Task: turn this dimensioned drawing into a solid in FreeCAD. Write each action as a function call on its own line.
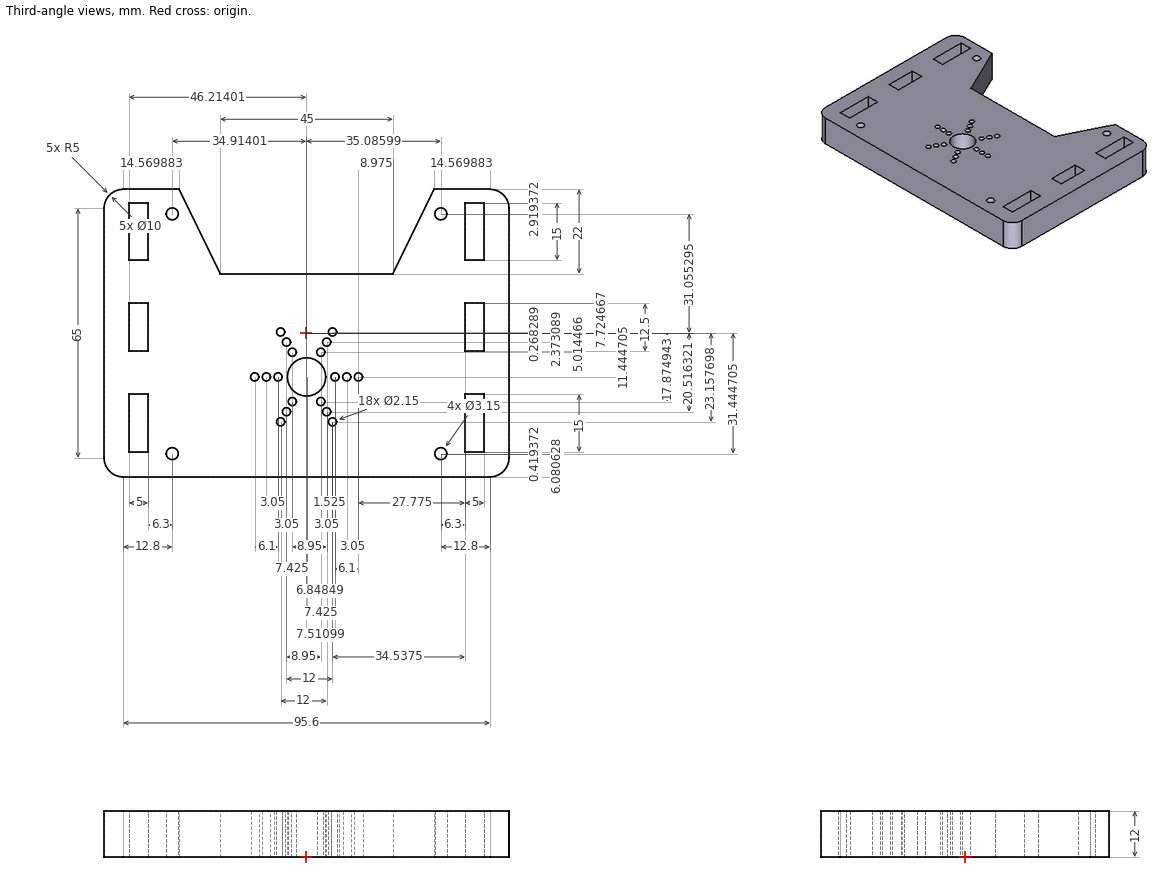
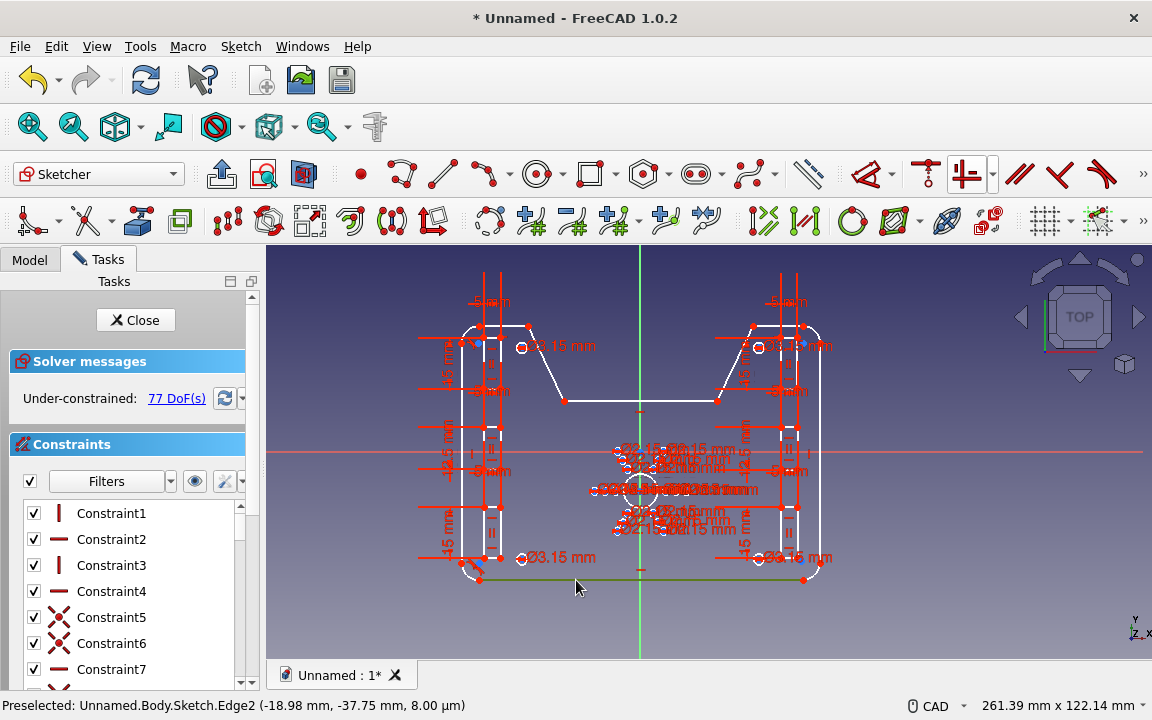
click(815, 575)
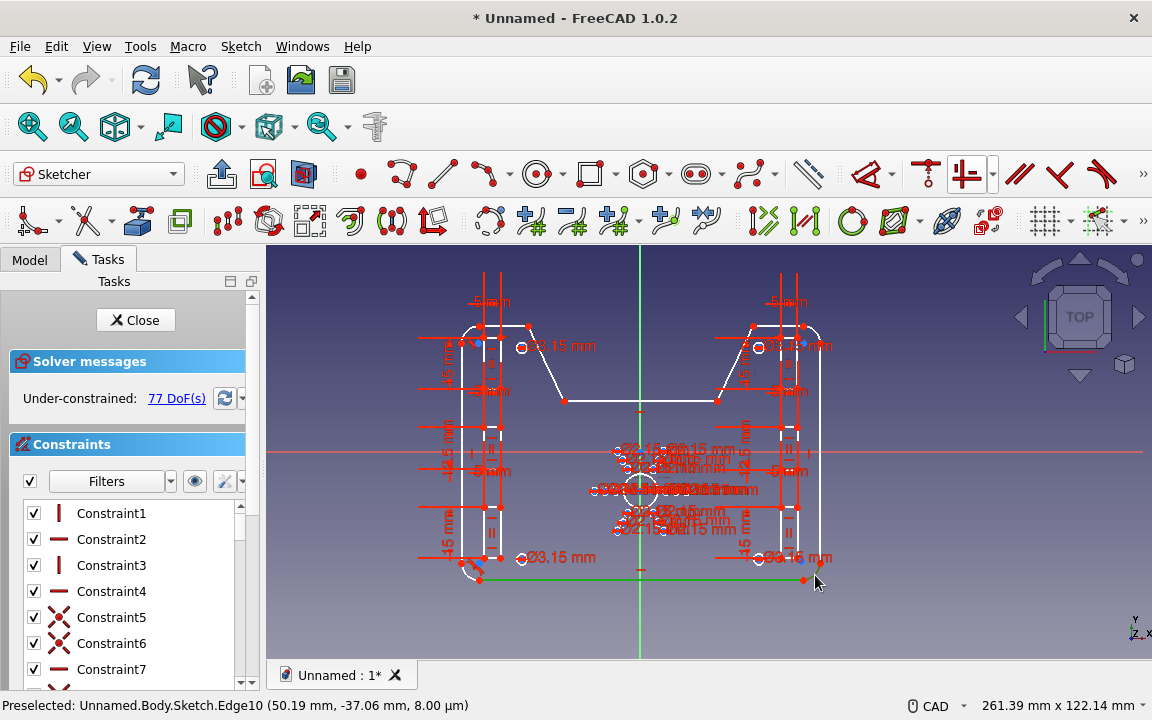
key(t)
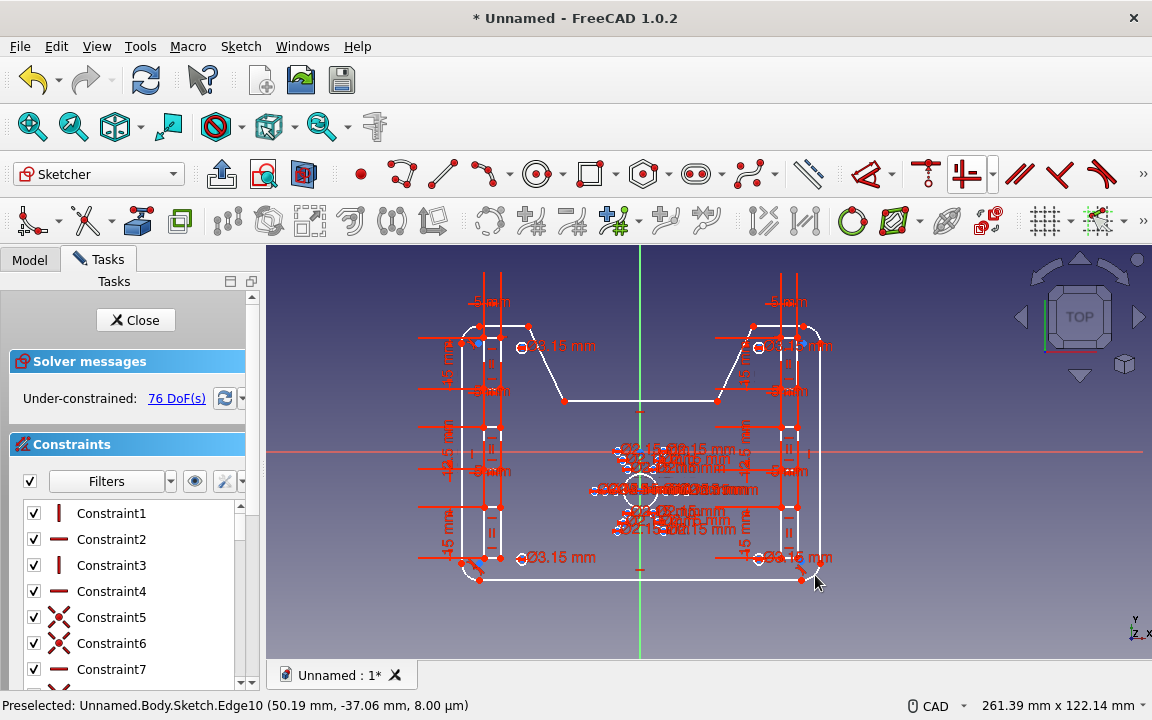
click(820, 497)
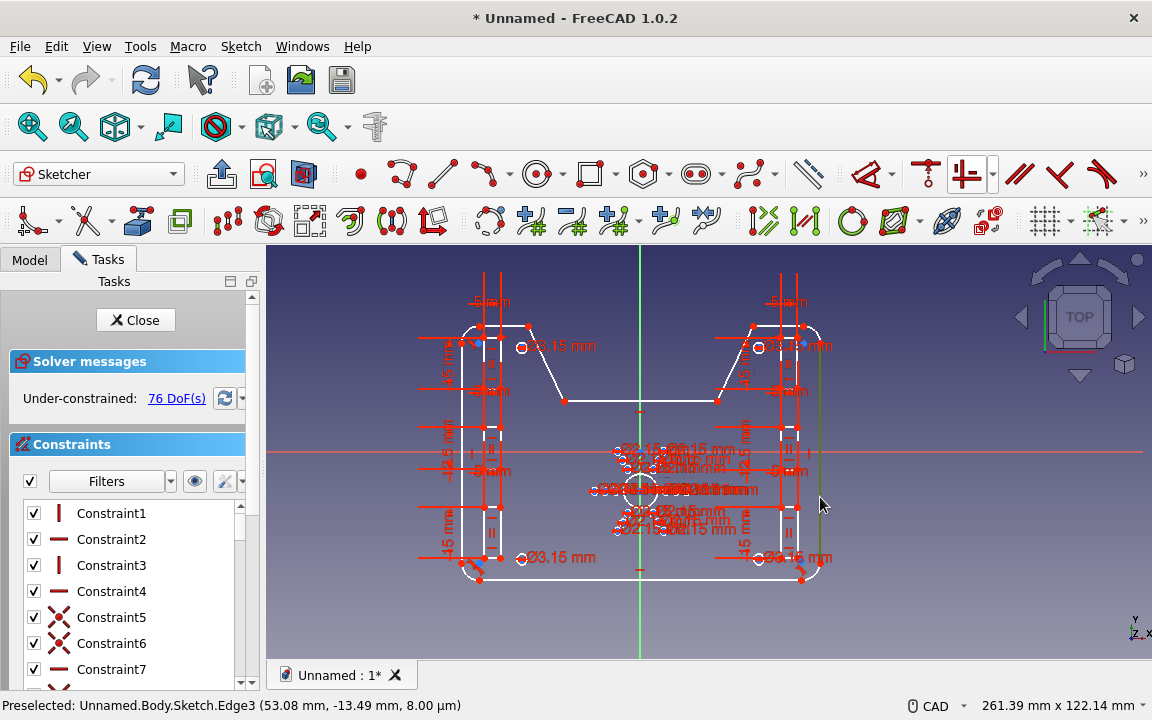
click(814, 575)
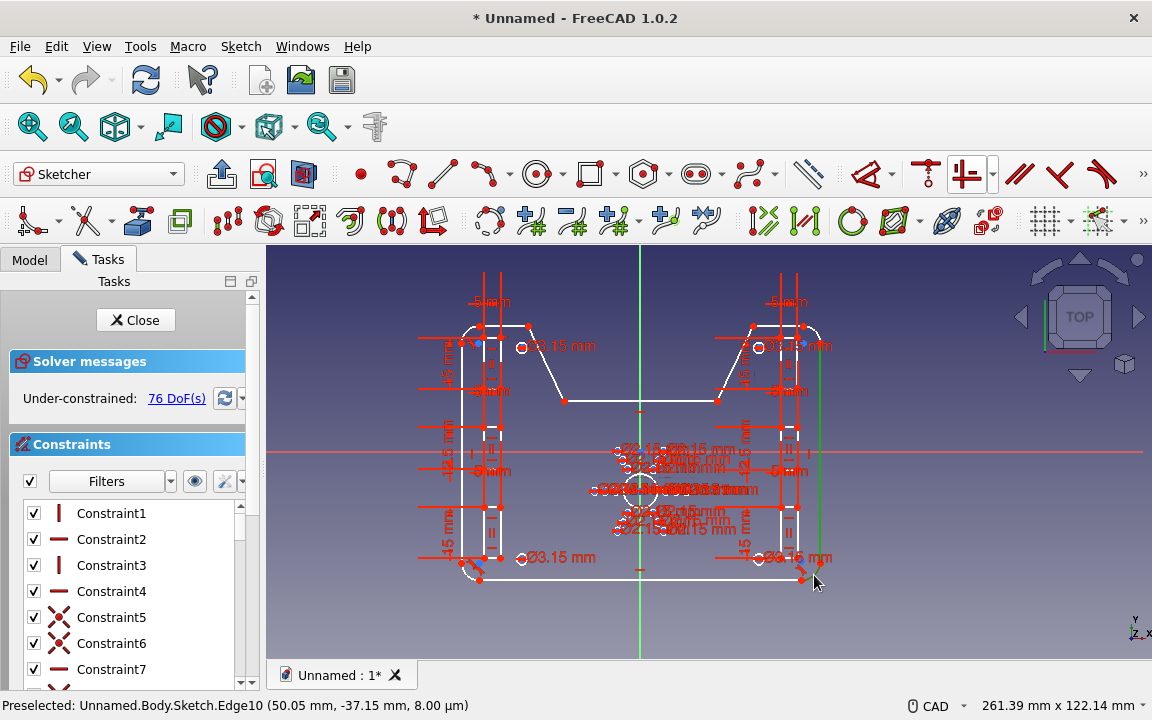
click(1102, 174)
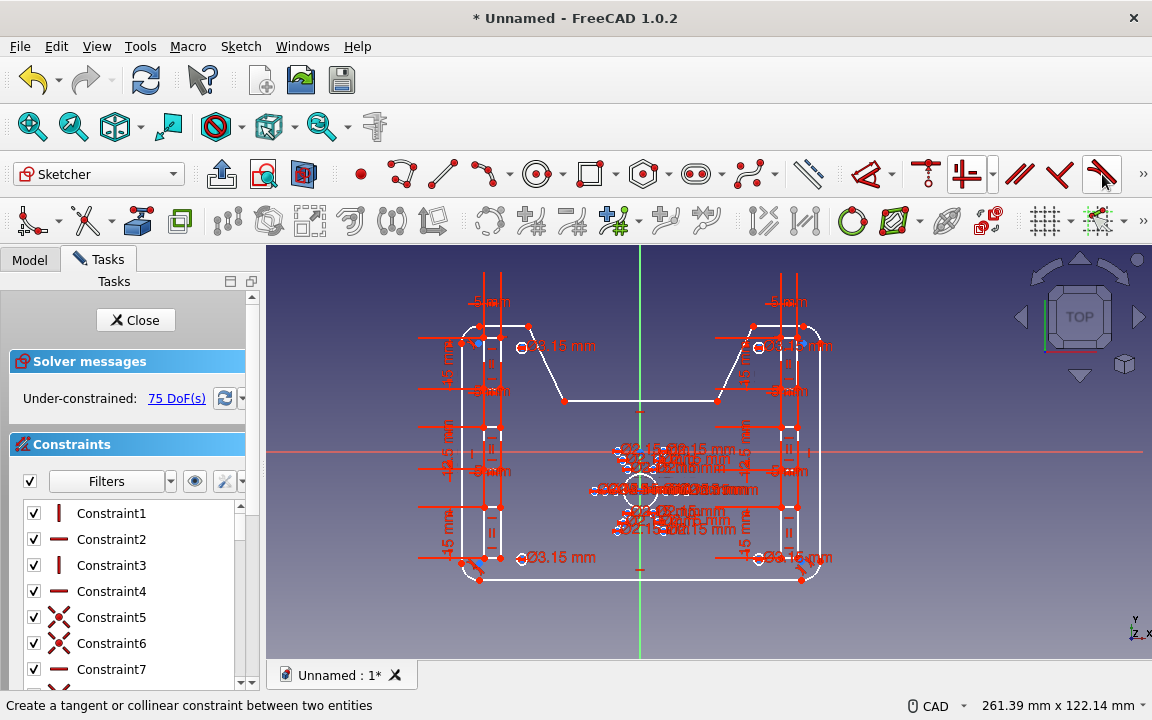
click(820, 496)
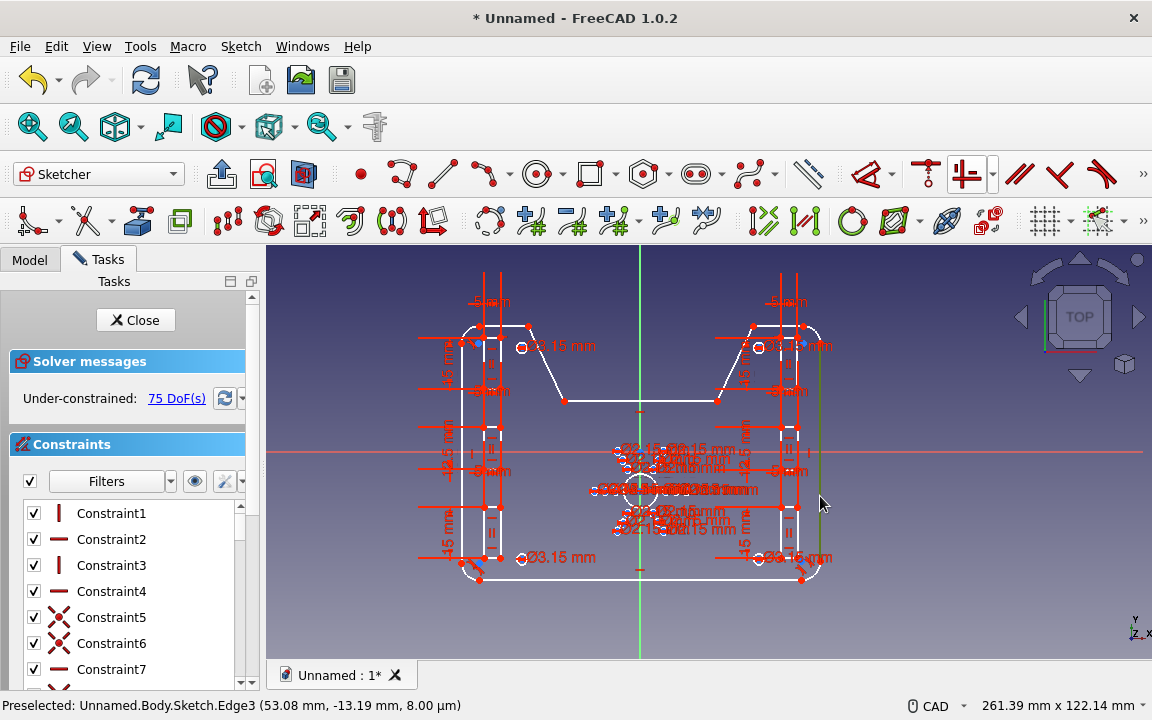
click(815, 331)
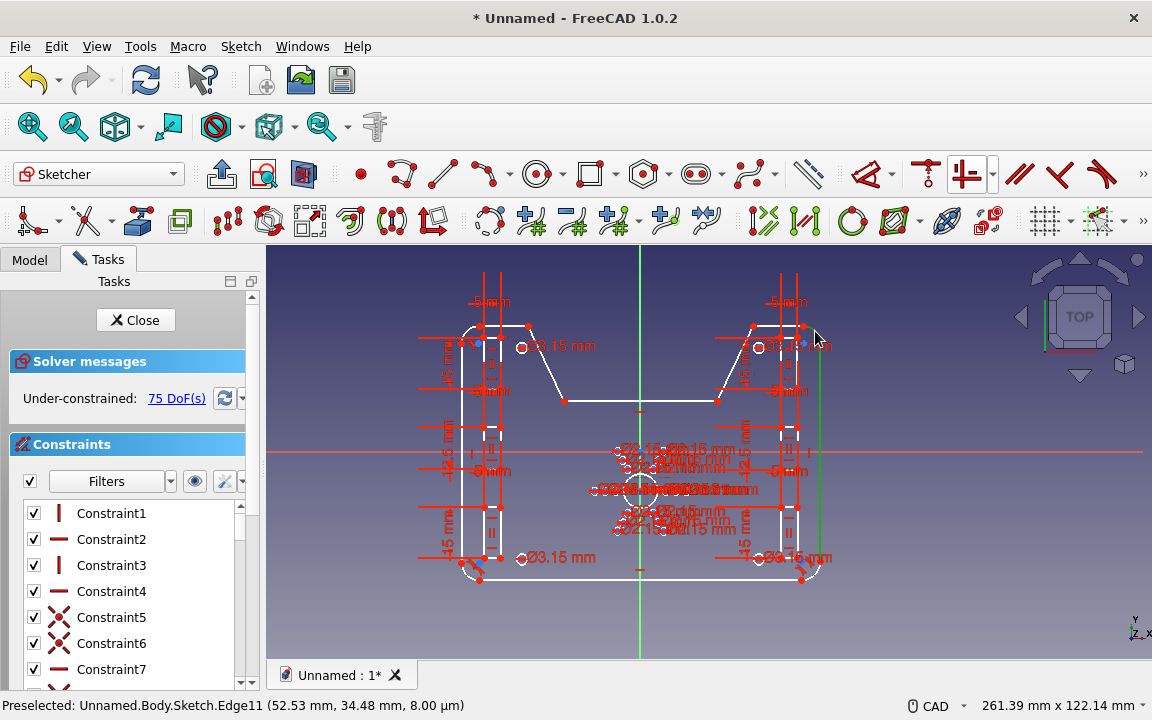
click(1102, 174)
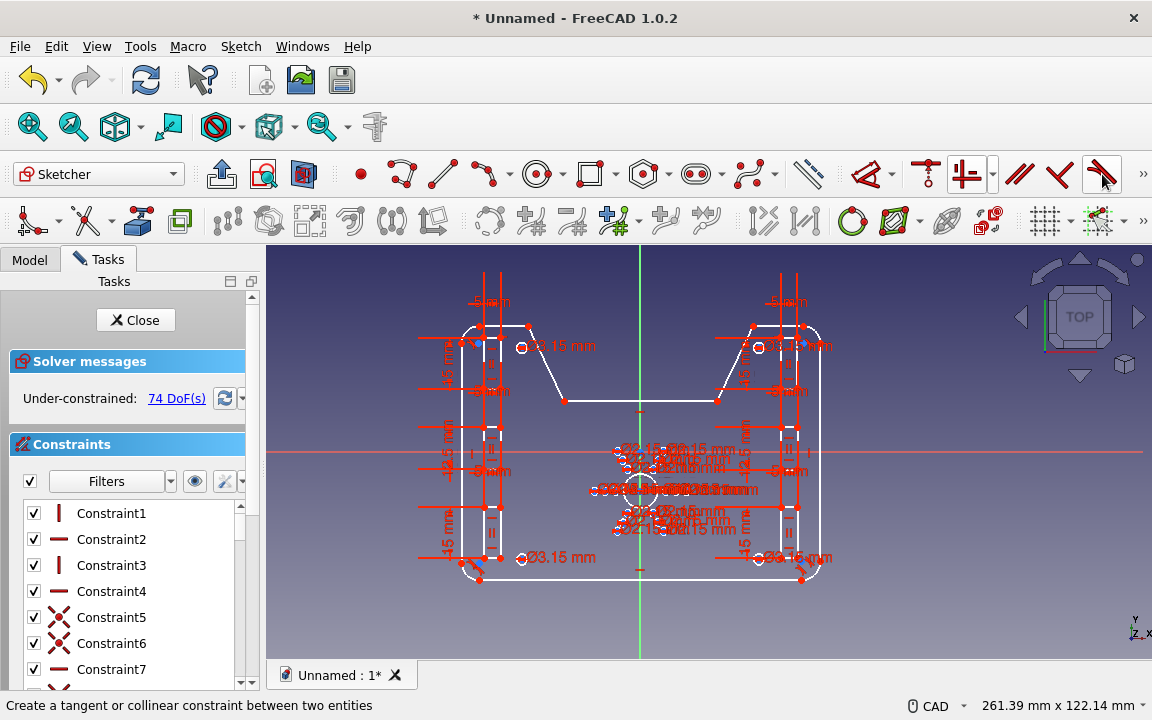
click(788, 326)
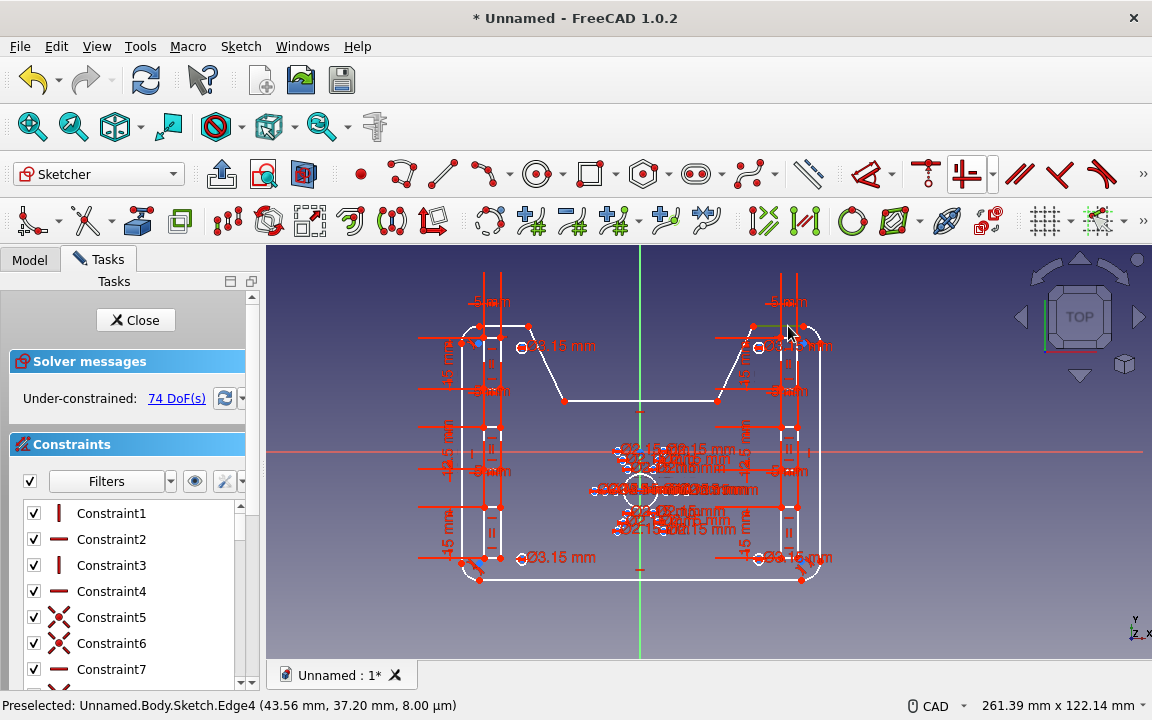
click(815, 331)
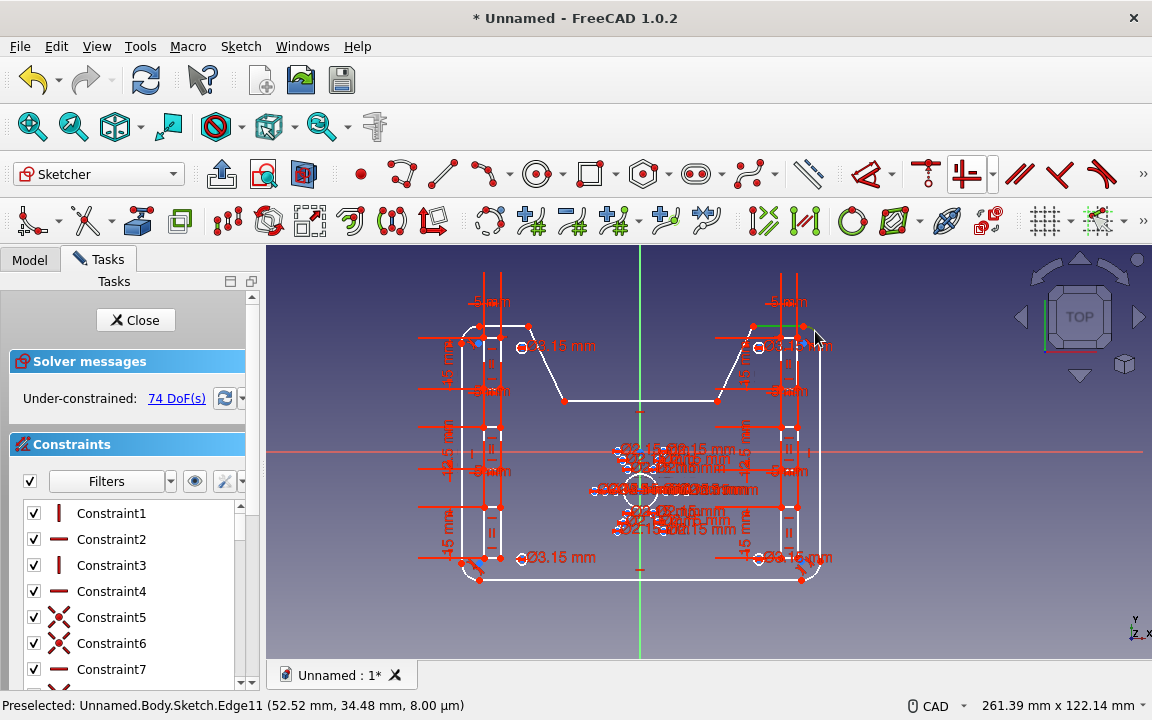
click(1102, 174)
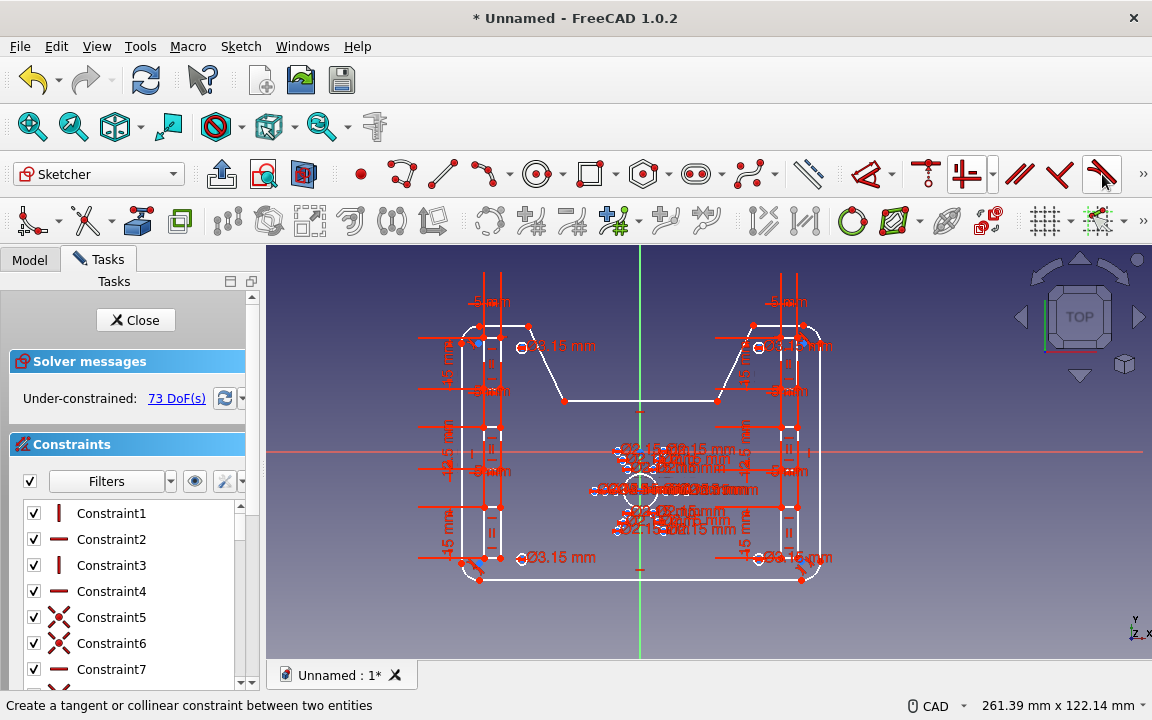
click(513, 326)